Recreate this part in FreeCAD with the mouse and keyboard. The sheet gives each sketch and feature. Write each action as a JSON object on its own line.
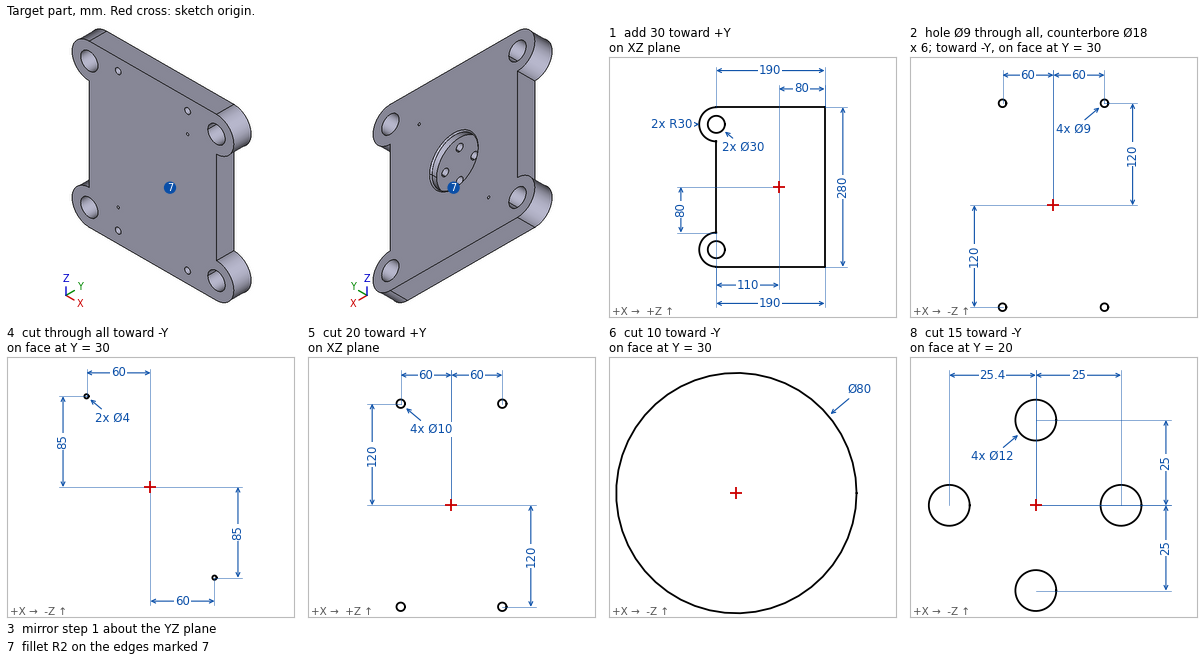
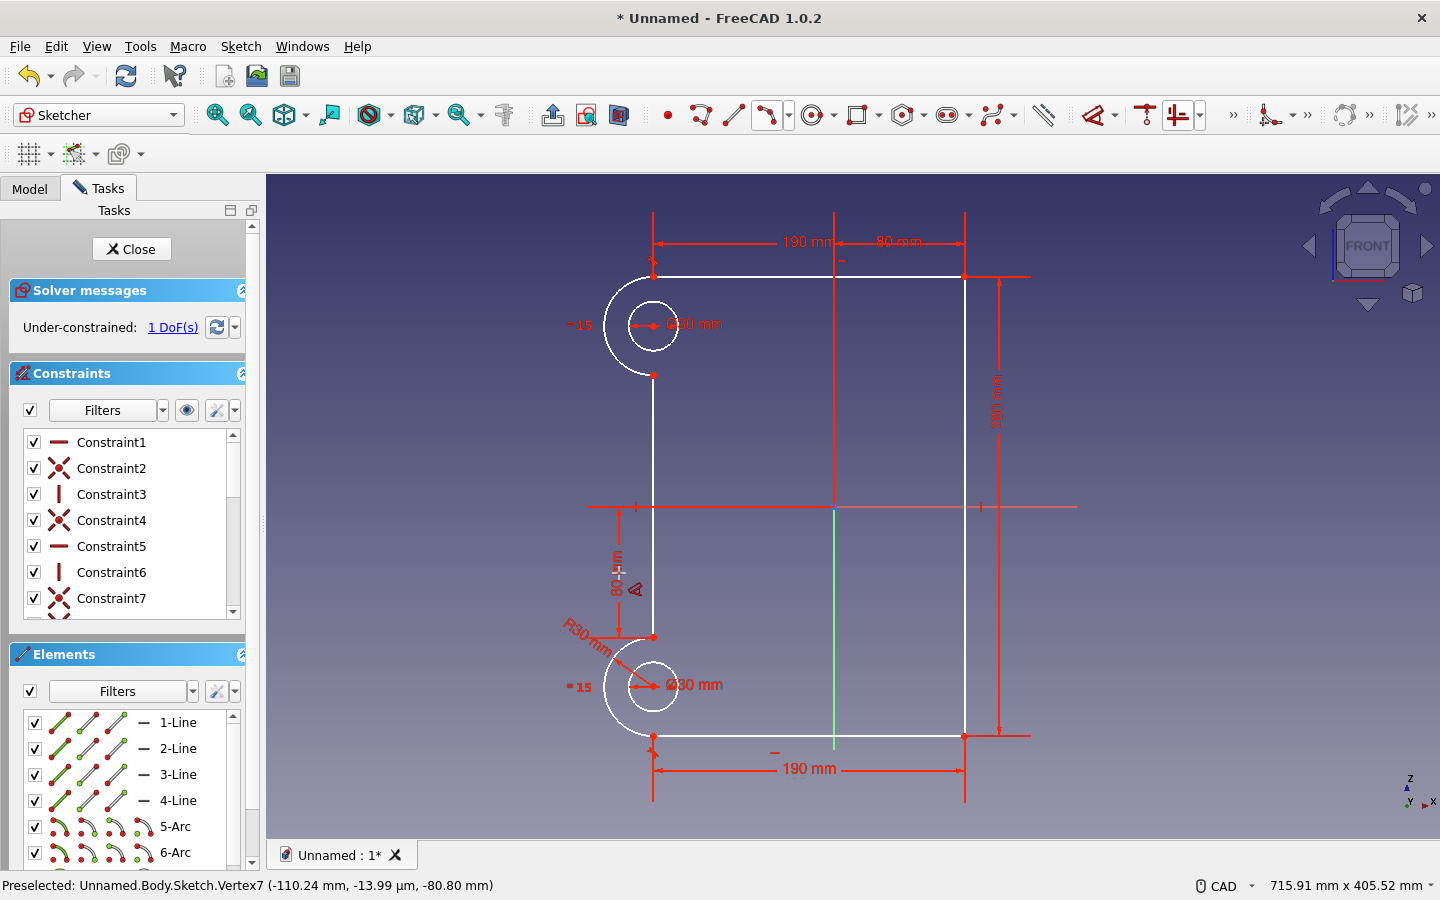
{"action": "left_click", "coordinate": [653, 638]}
{"action": "left_click", "coordinate": [743, 672]}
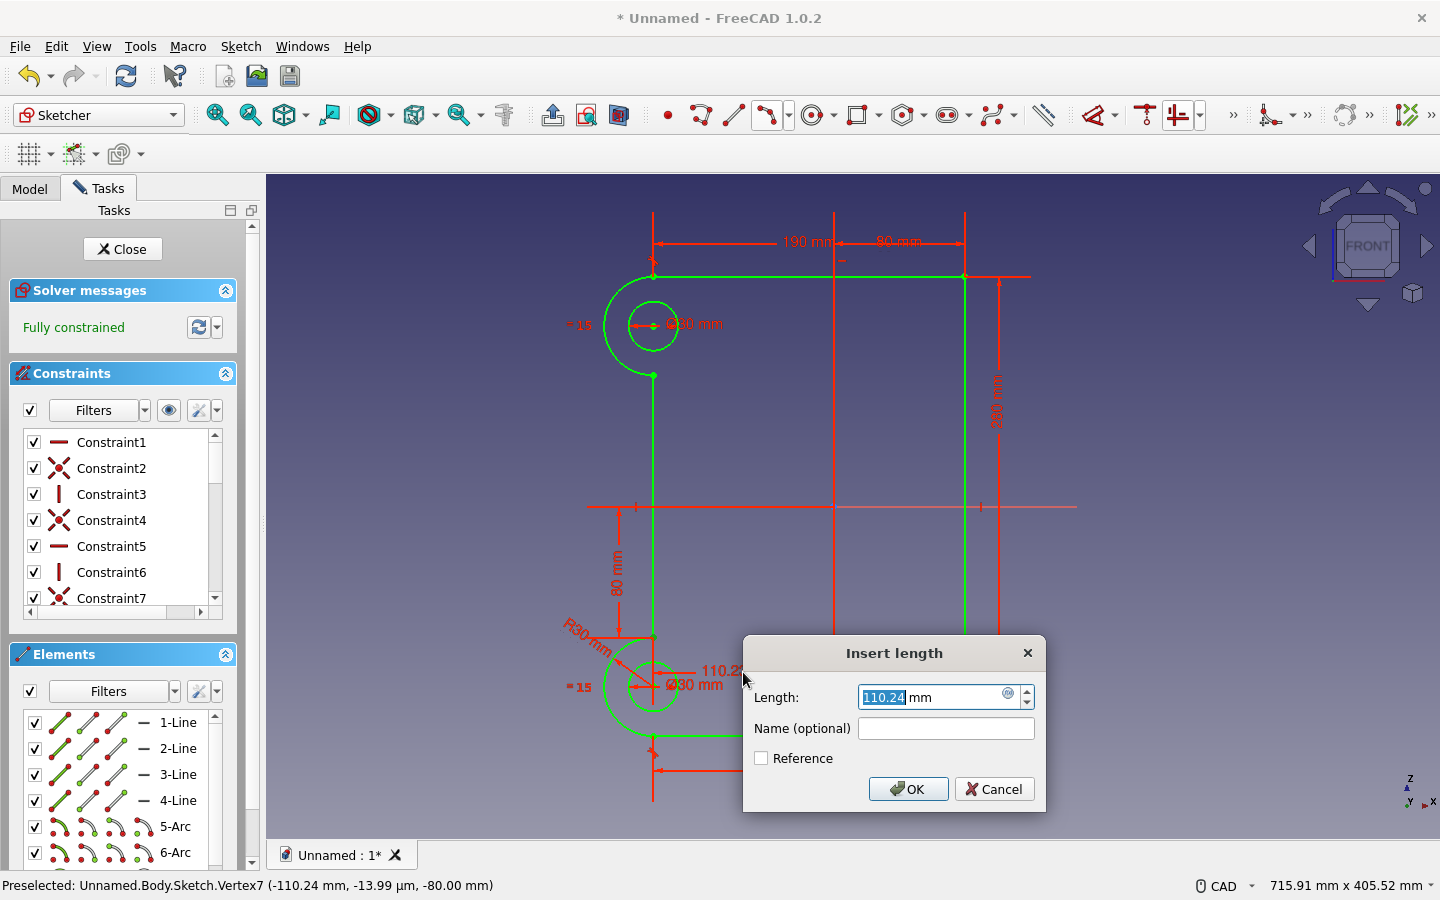
{"action": "type", "text": "110"}
{"action": "key", "text": "Return"}
{"action": "key", "text": "Escape"}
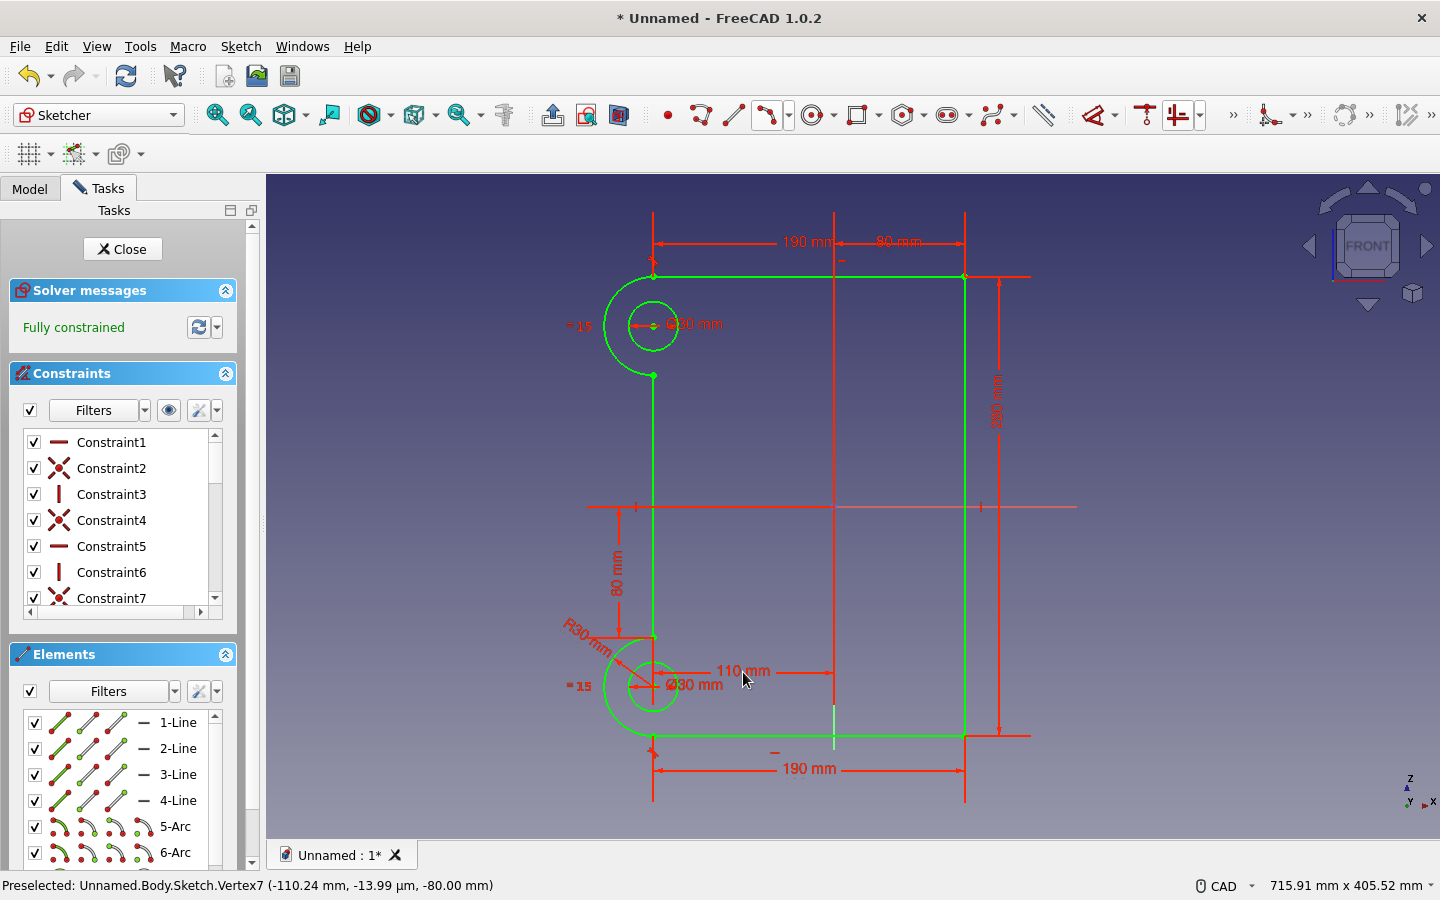
{"action": "left_click", "coordinate": [123, 249]}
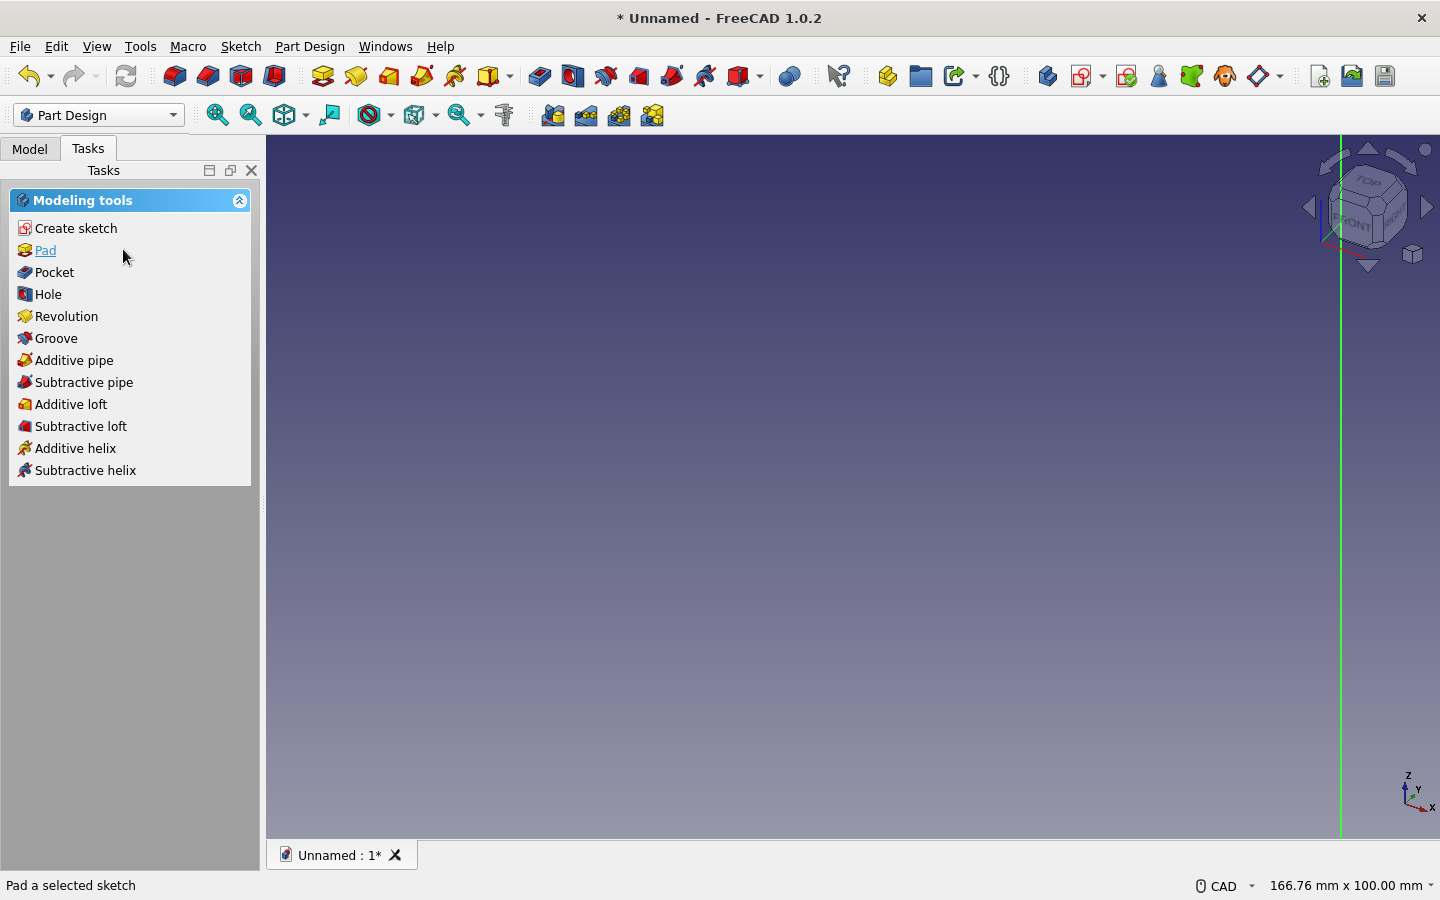
{"action": "left_click", "coordinate": [323, 76]}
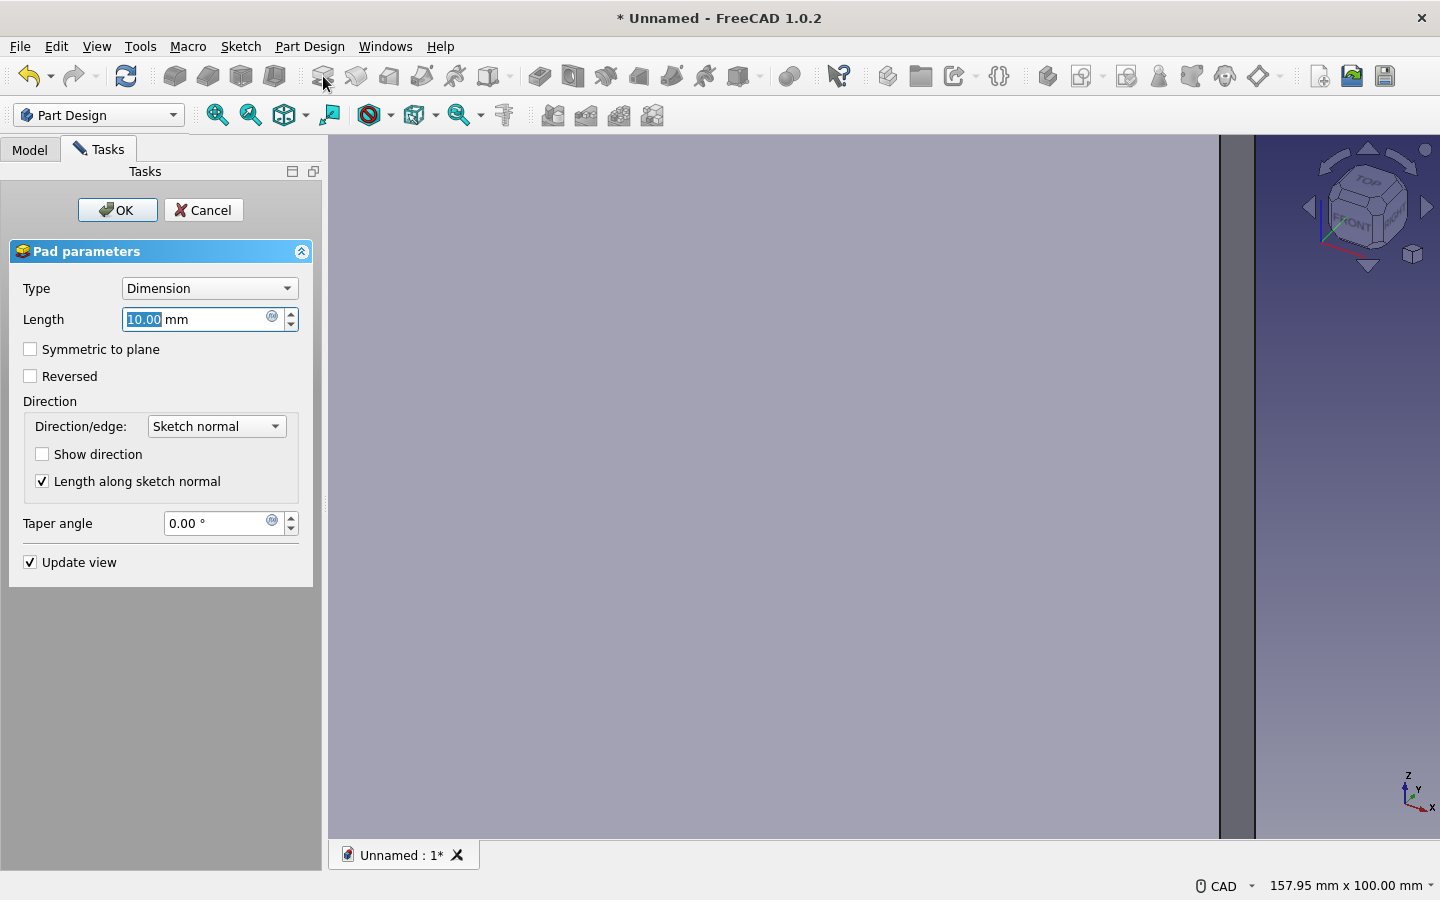
{"action": "type", "text": "30"}
{"action": "key", "text": "Tab"}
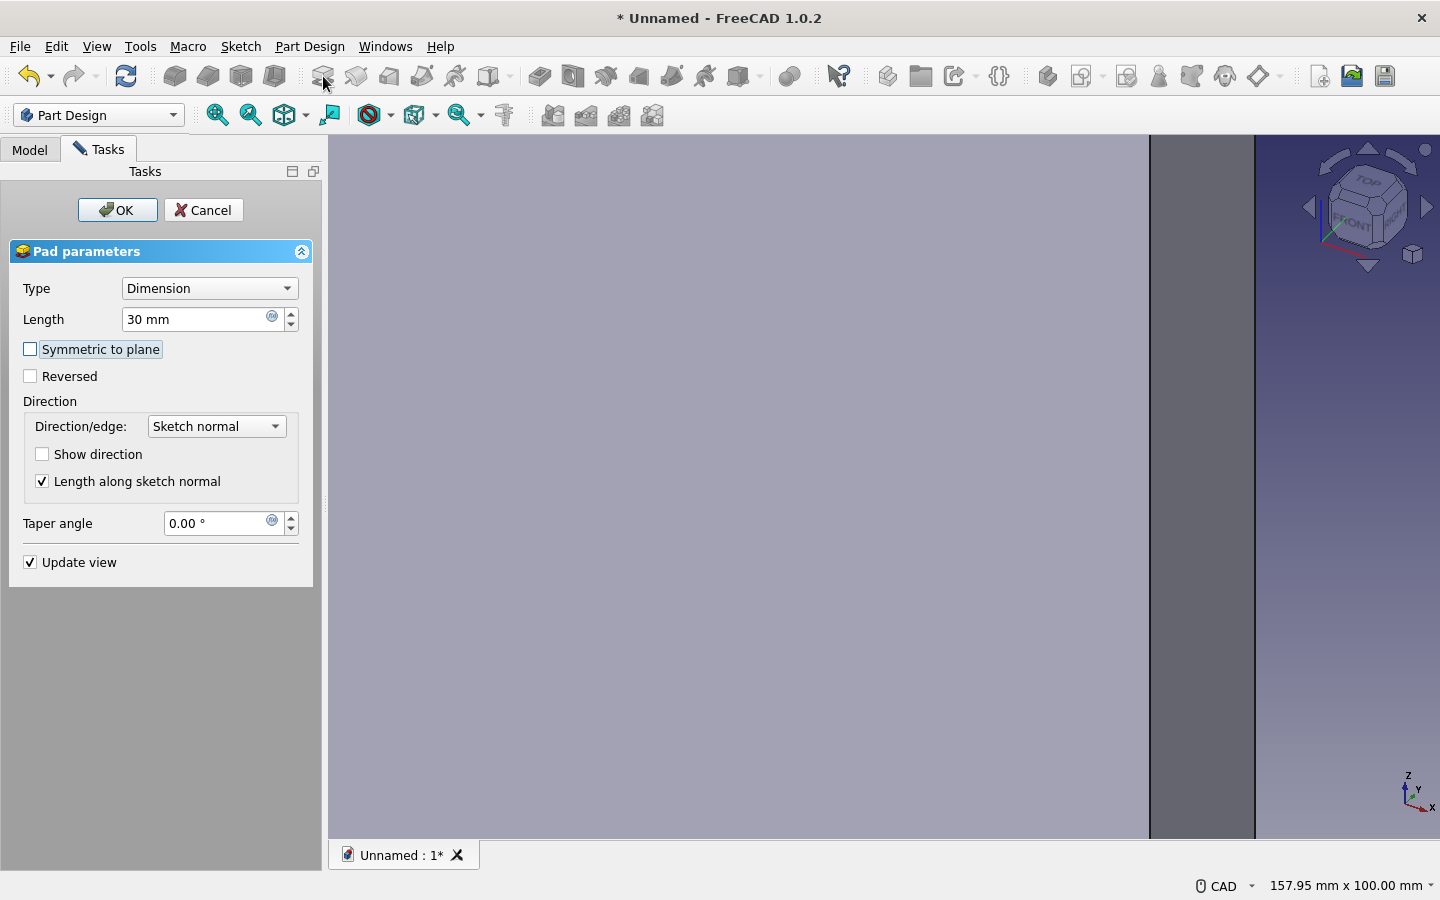
{"action": "left_click", "coordinate": [31, 376]}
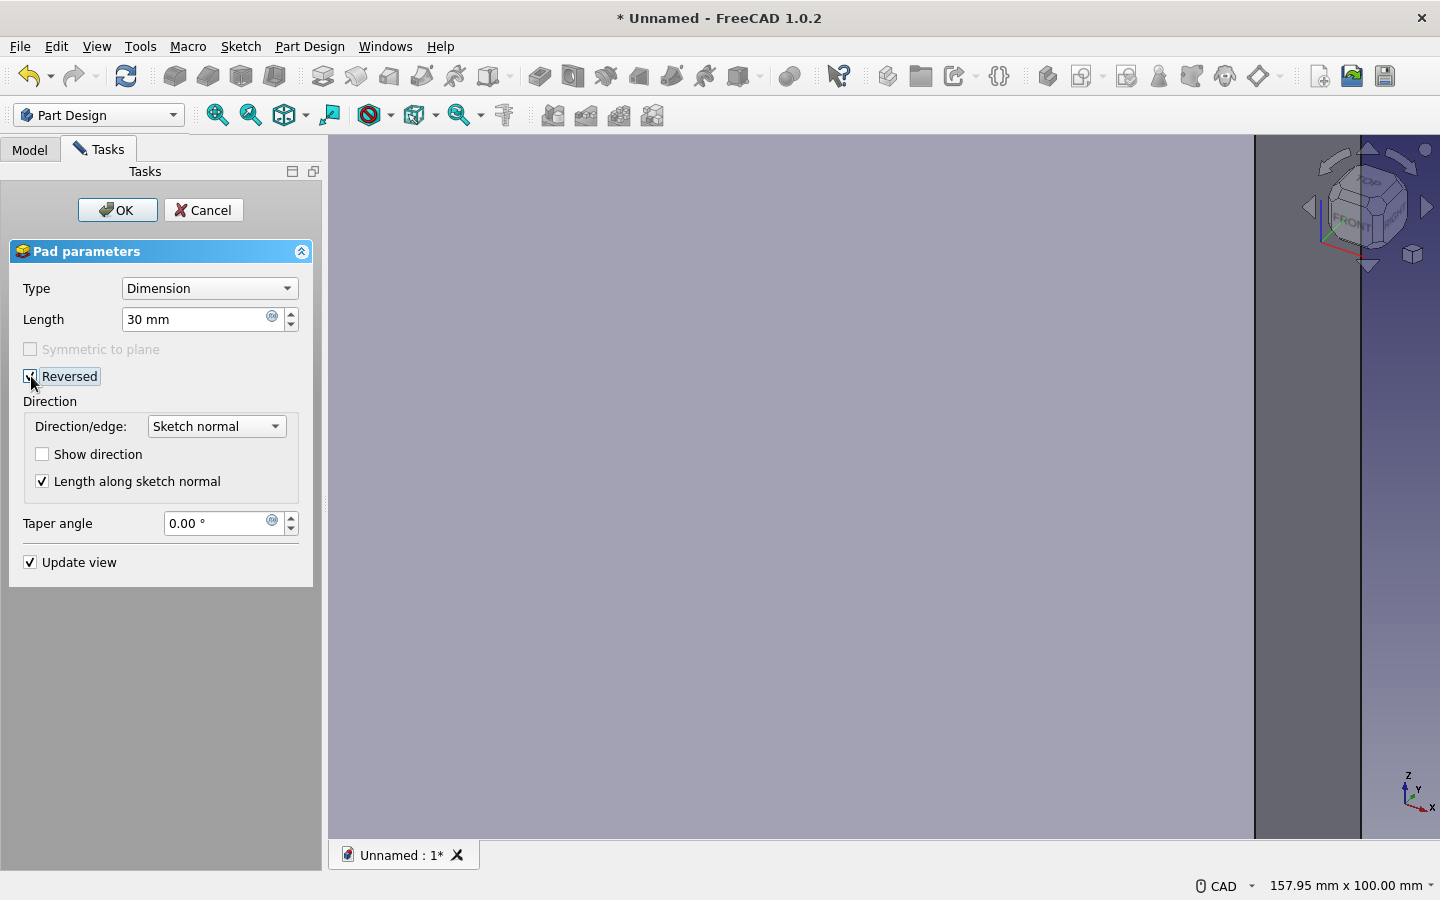
{"action": "left_click", "coordinate": [118, 210]}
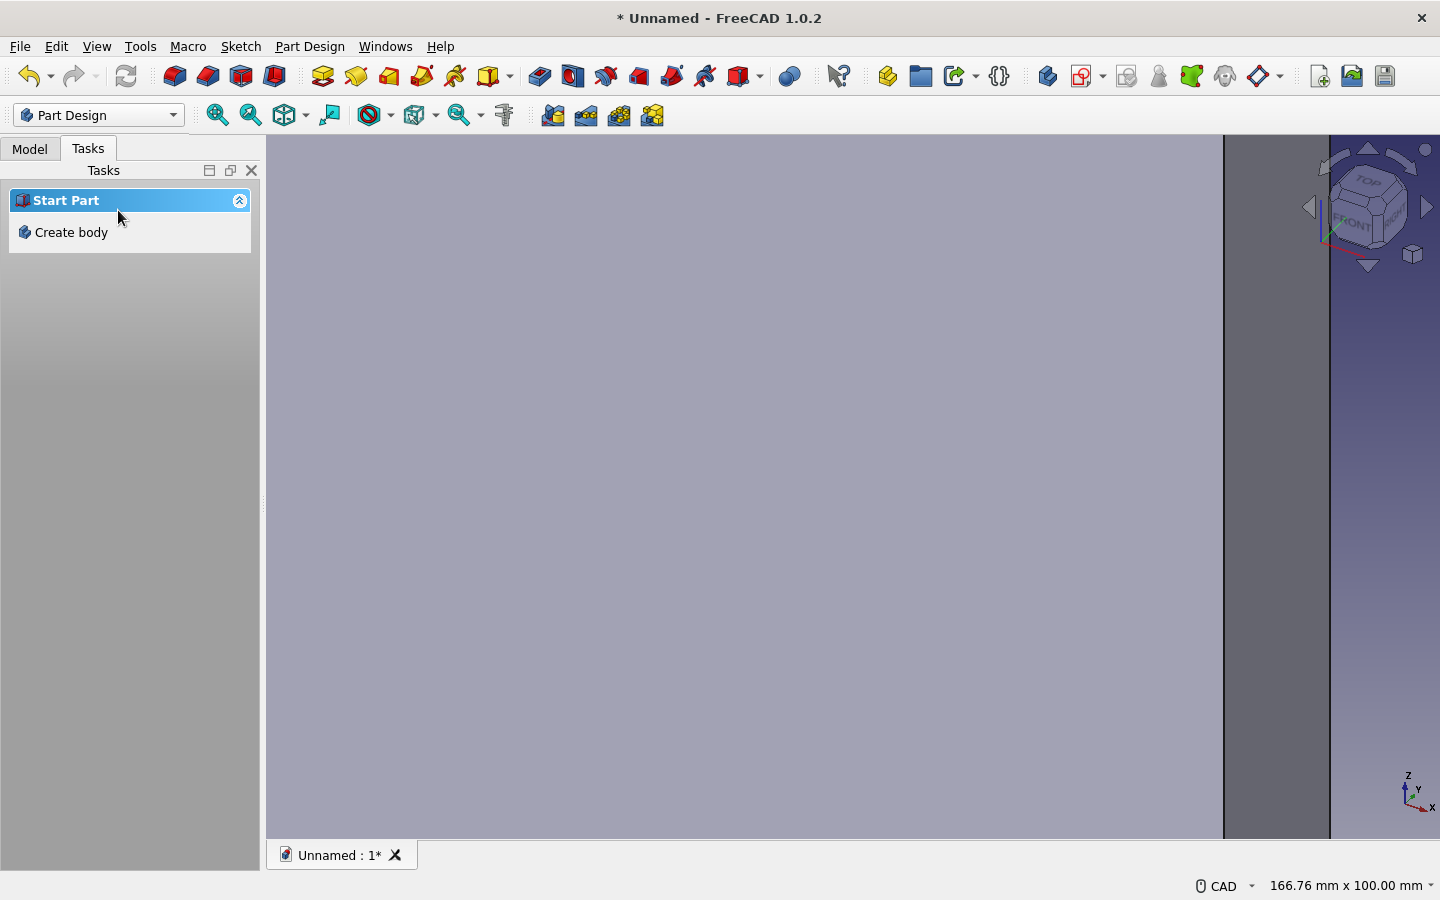
{"action": "left_click", "coordinate": [218, 116]}